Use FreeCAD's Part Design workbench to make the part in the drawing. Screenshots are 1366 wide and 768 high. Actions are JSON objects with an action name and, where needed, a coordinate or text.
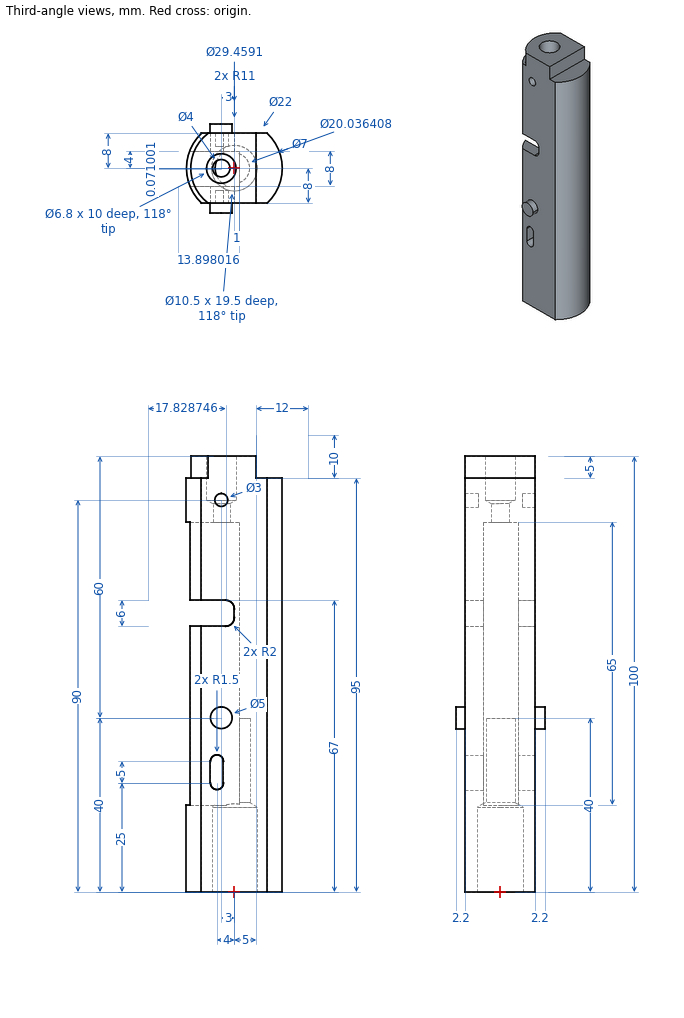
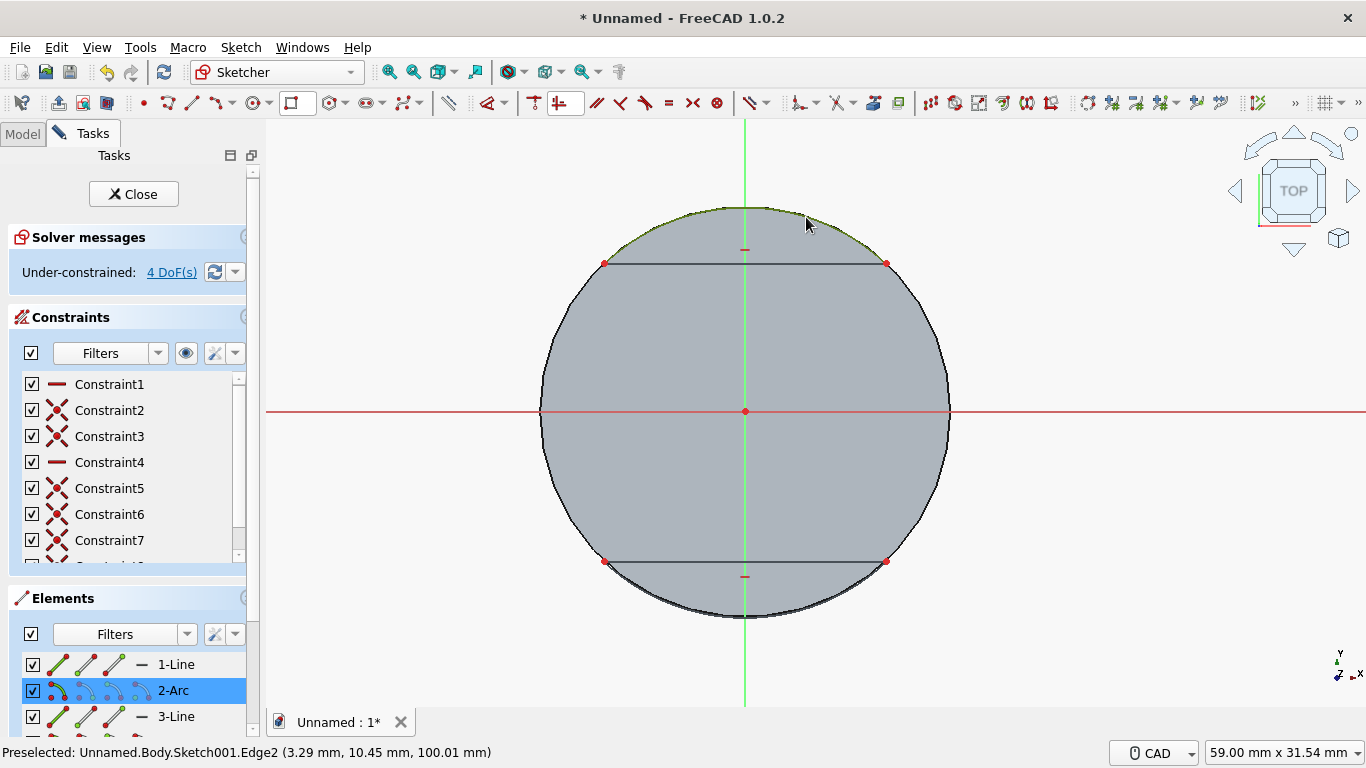
{"action": "left_click", "coordinate": [684, 609]}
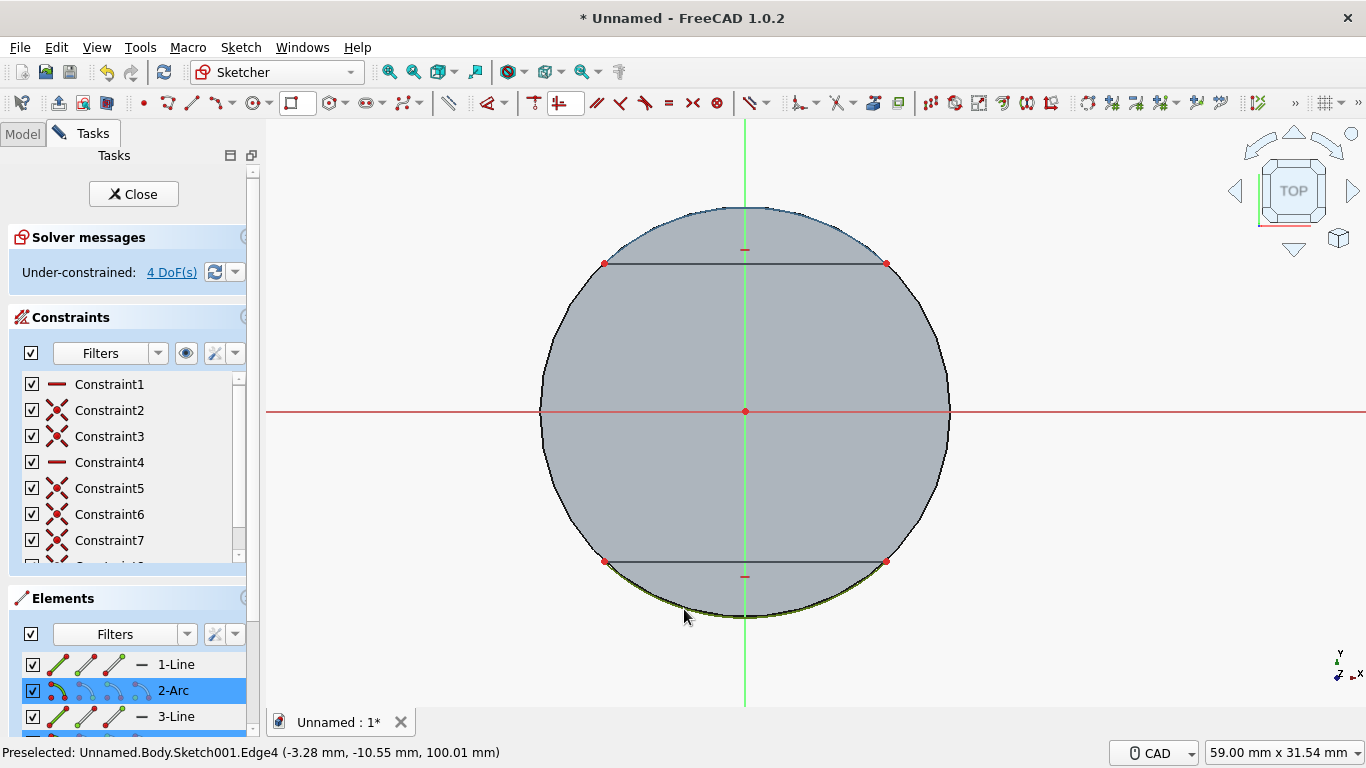
{"action": "left_click", "coordinate": [670, 104]}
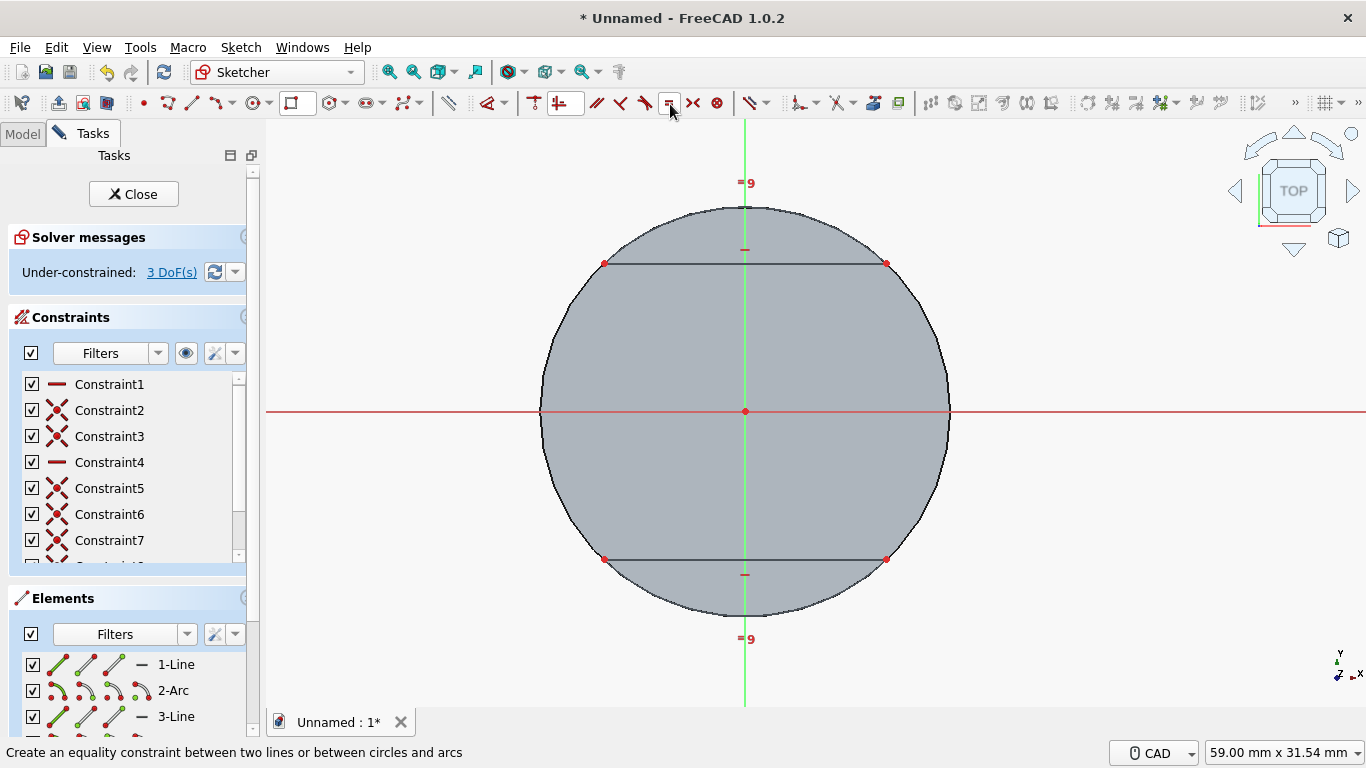
{"action": "left_click", "coordinate": [488, 104]}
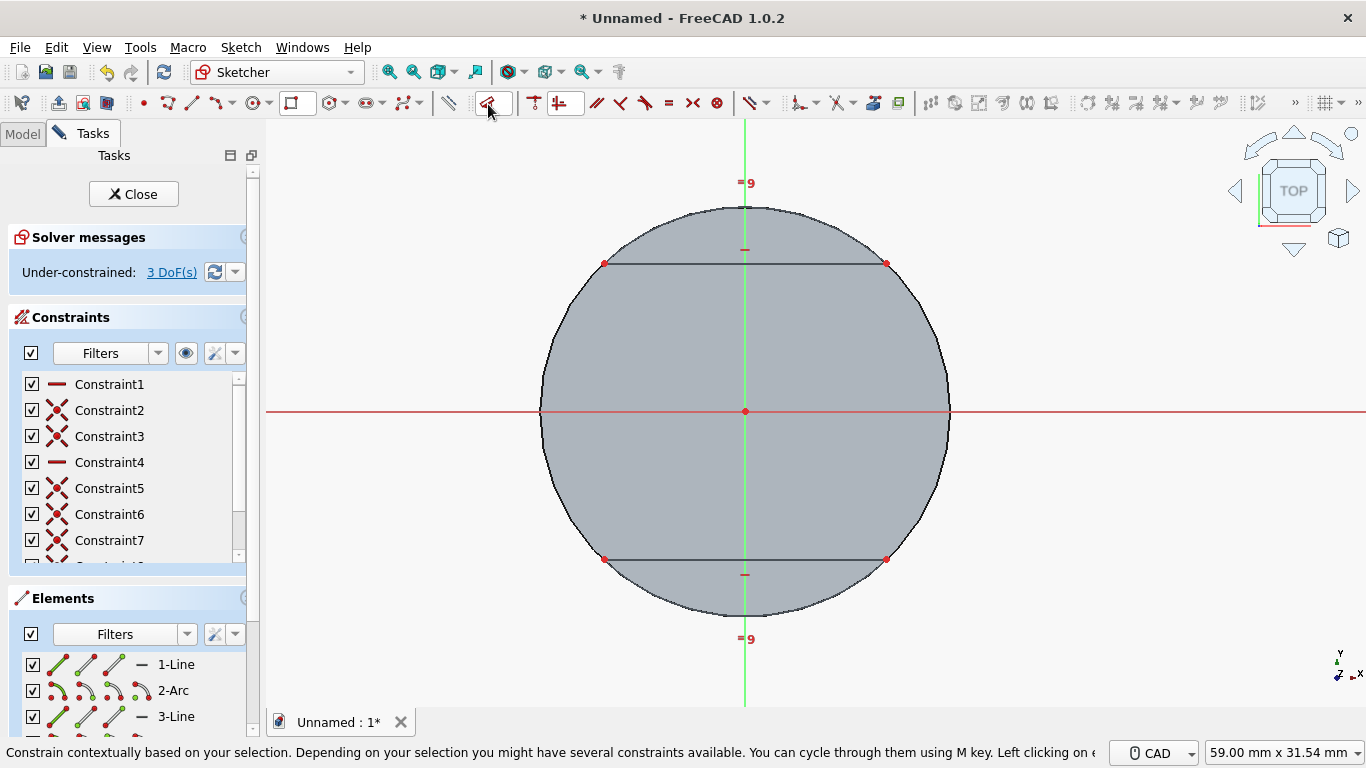
{"action": "left_click", "coordinate": [806, 217]}
{"action": "left_click", "coordinate": [816, 186]}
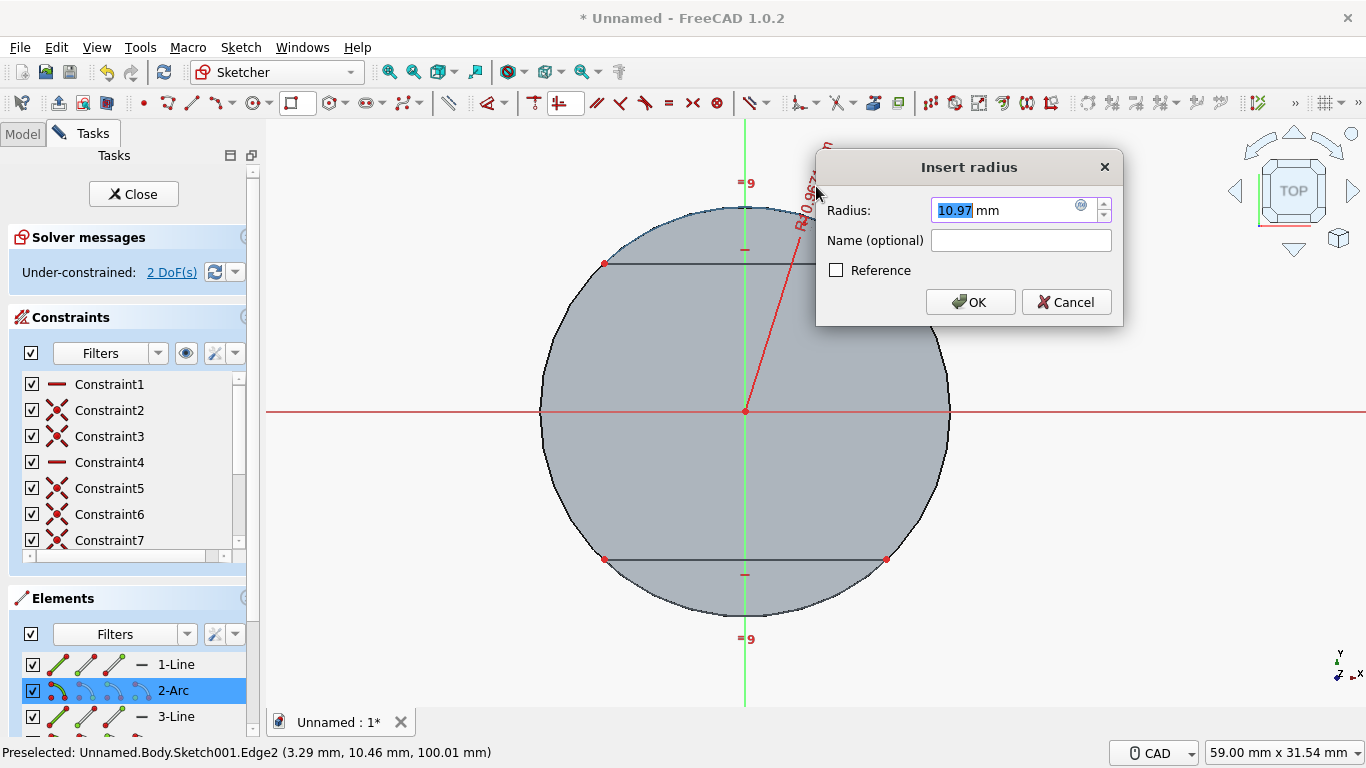
{"action": "type", "text": "11"}
{"action": "key", "text": "Return"}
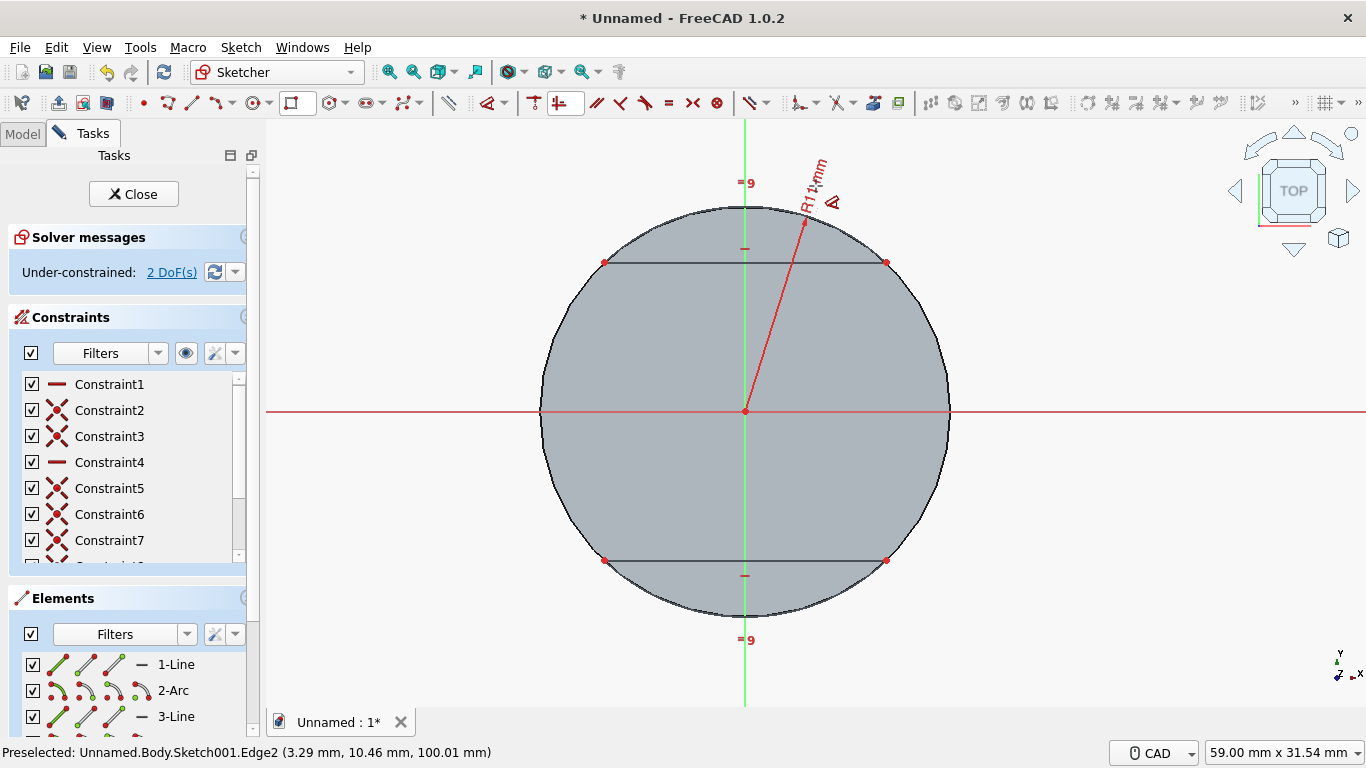
{"action": "left_click", "coordinate": [604, 263]}
{"action": "left_click", "coordinate": [570, 337]}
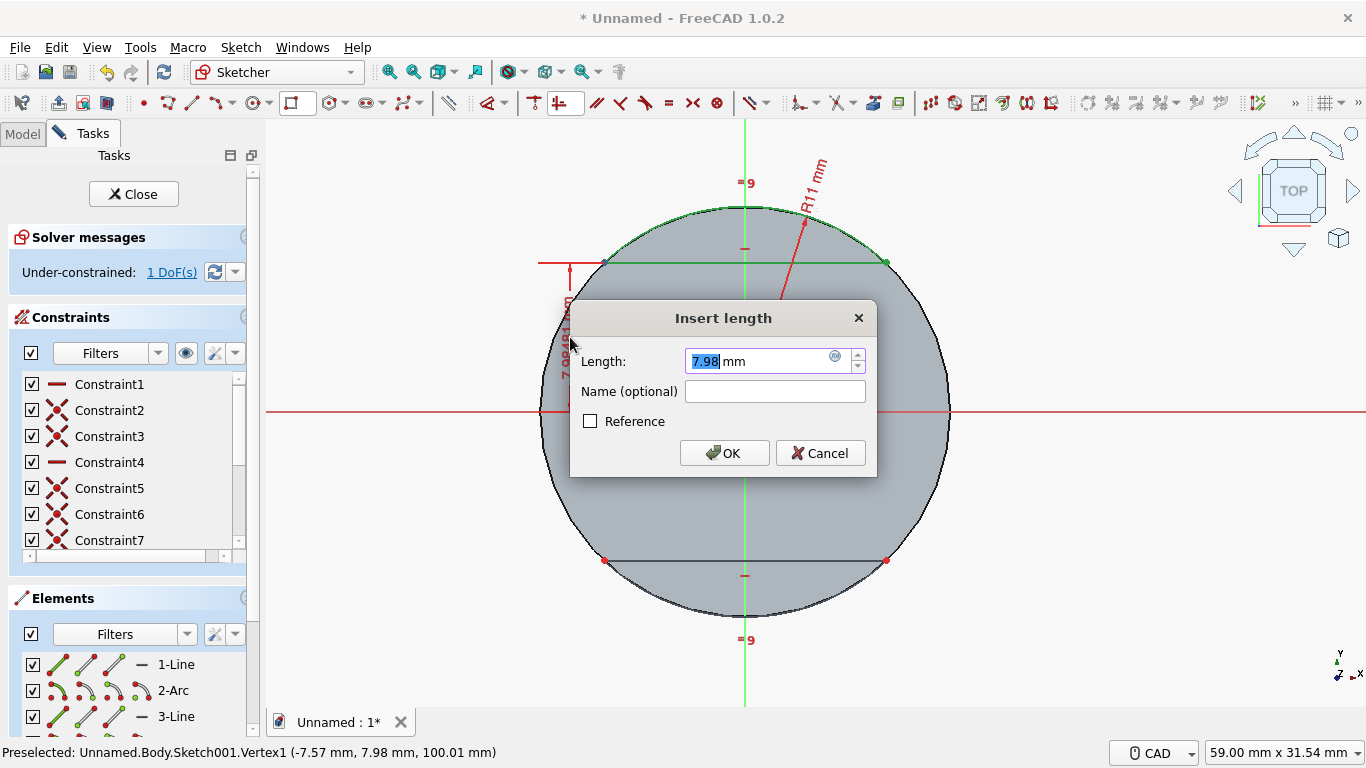
{"action": "type", "text": "8"}
{"action": "key", "text": "Return"}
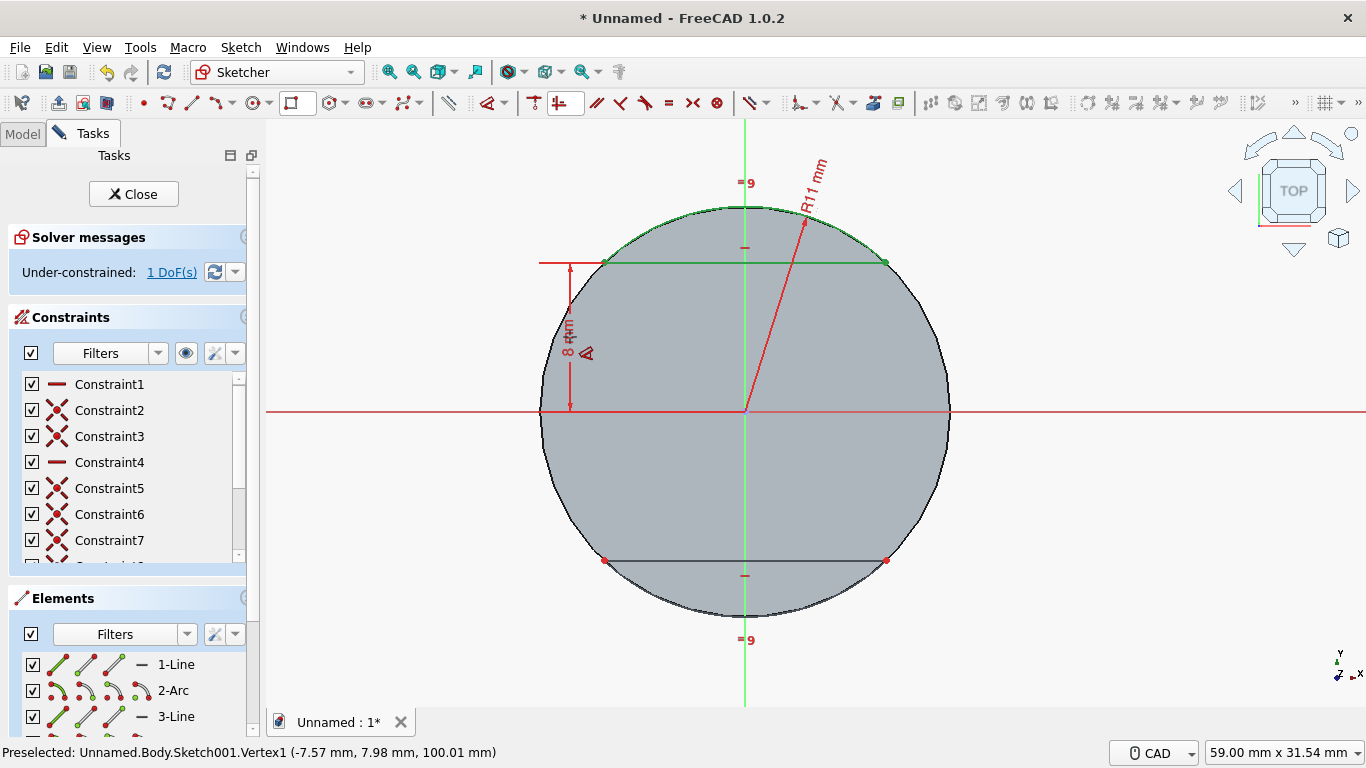
{"action": "left_click", "coordinate": [886, 561]}
{"action": "left_click", "coordinate": [920, 486]}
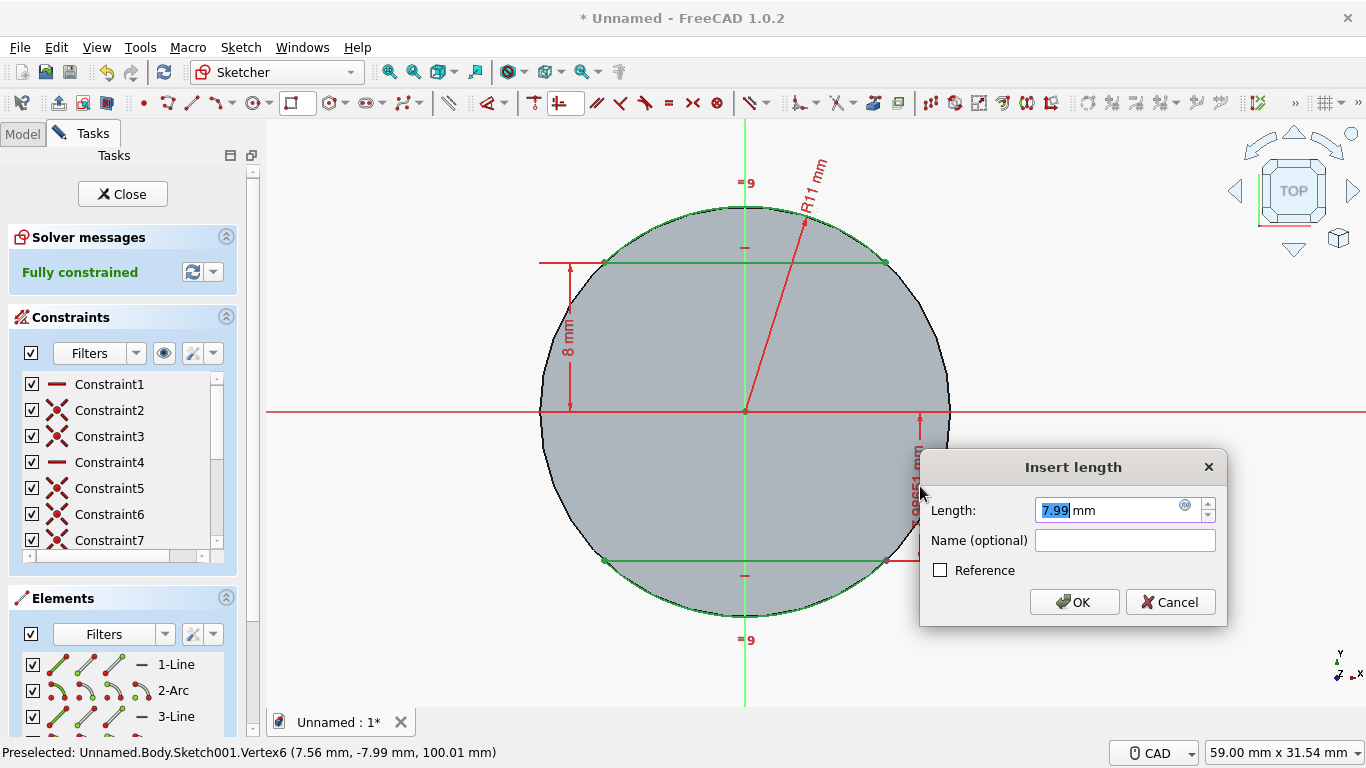
{"action": "type", "text": "8"}
{"action": "key", "text": "Return"}
{"action": "key", "text": "Escape"}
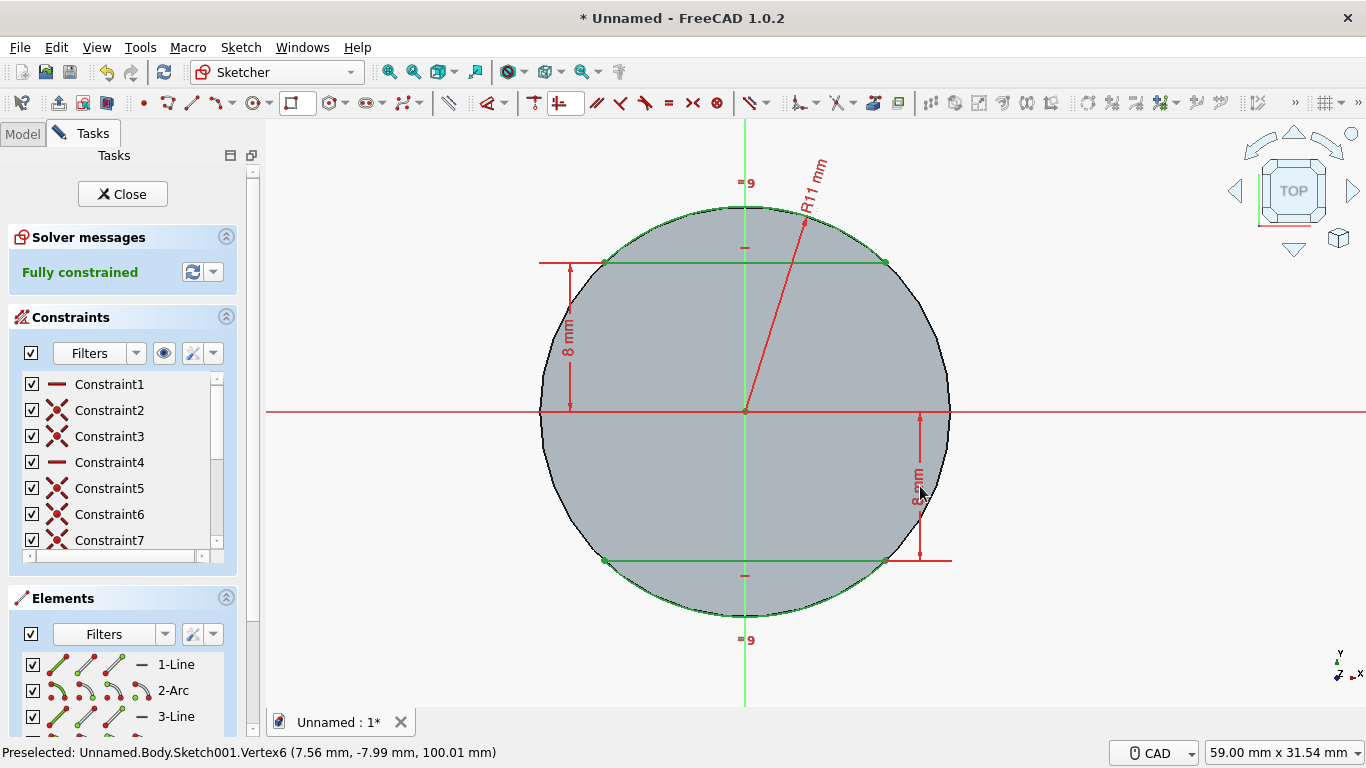
{"action": "left_click", "coordinate": [123, 194]}